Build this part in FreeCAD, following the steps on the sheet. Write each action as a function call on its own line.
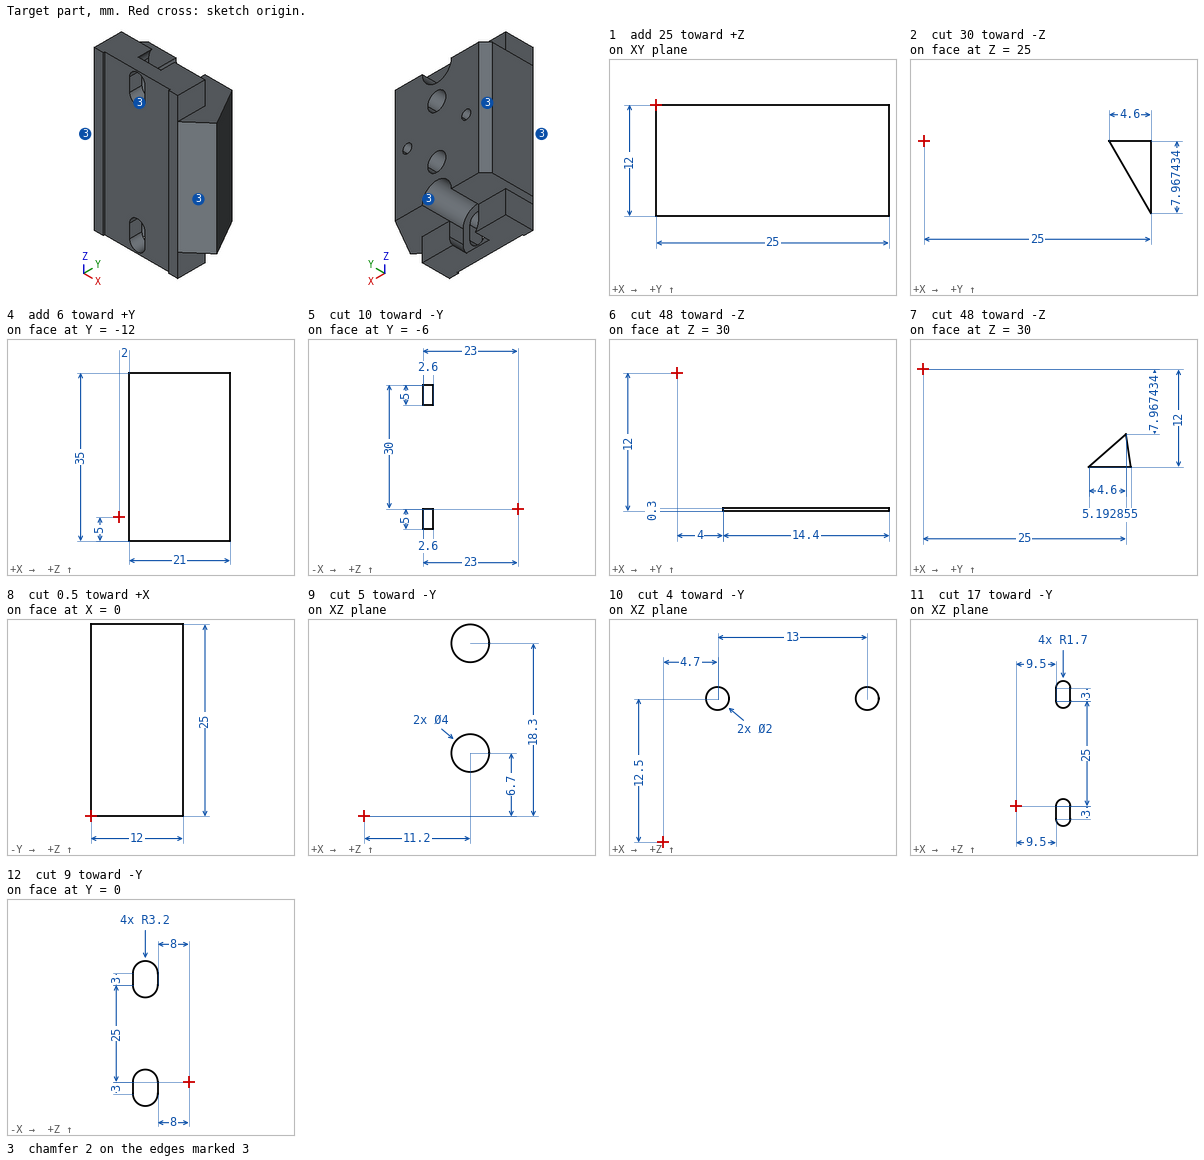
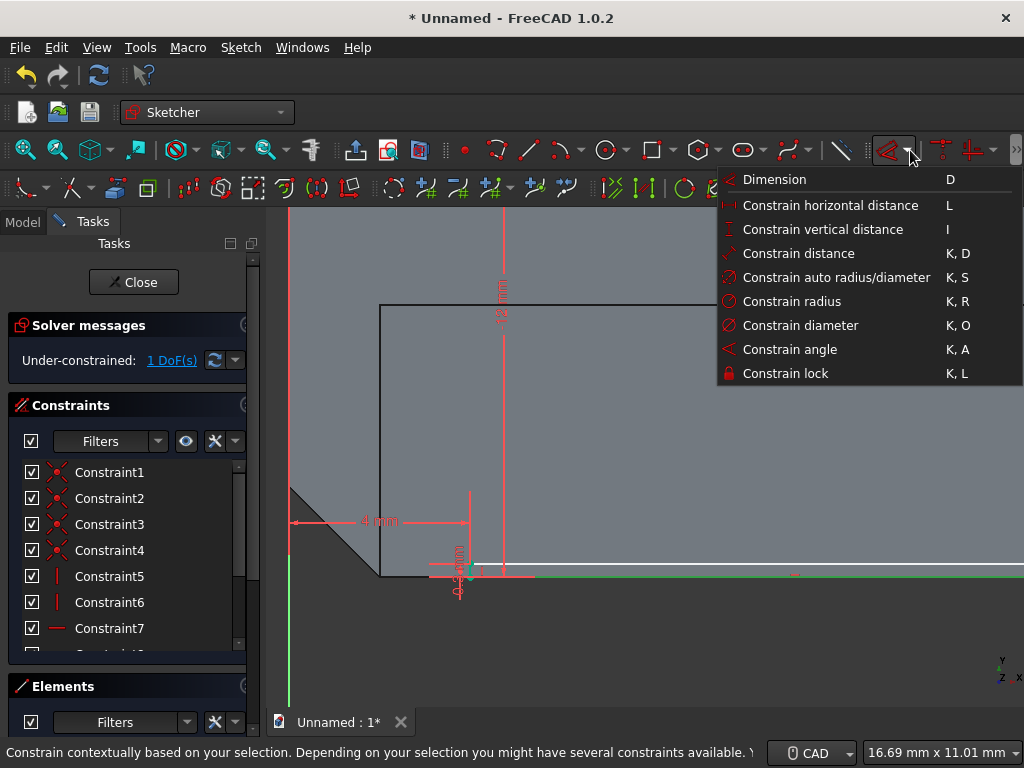
click(870, 205)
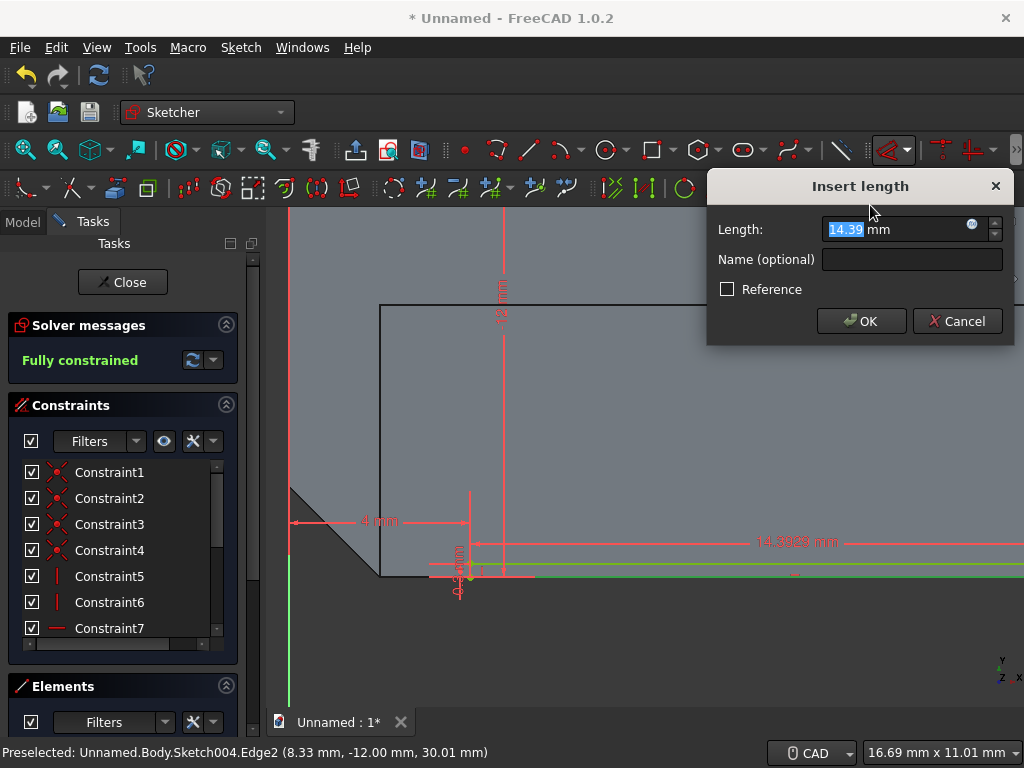
text(14.4)
key(Return)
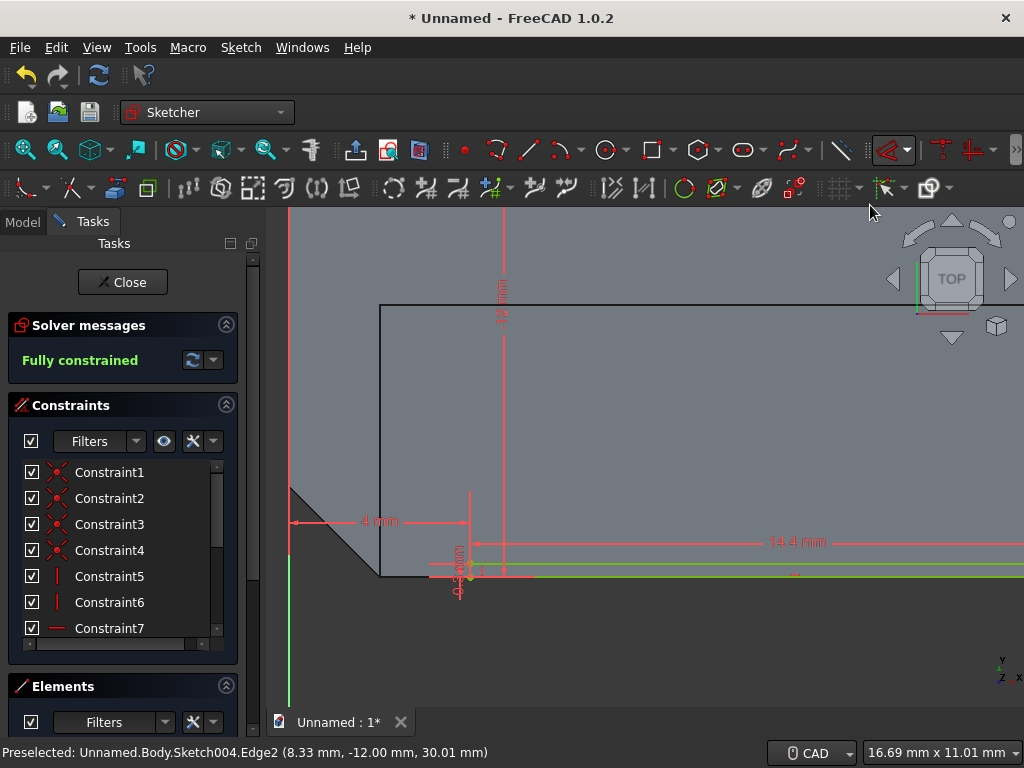
click(123, 282)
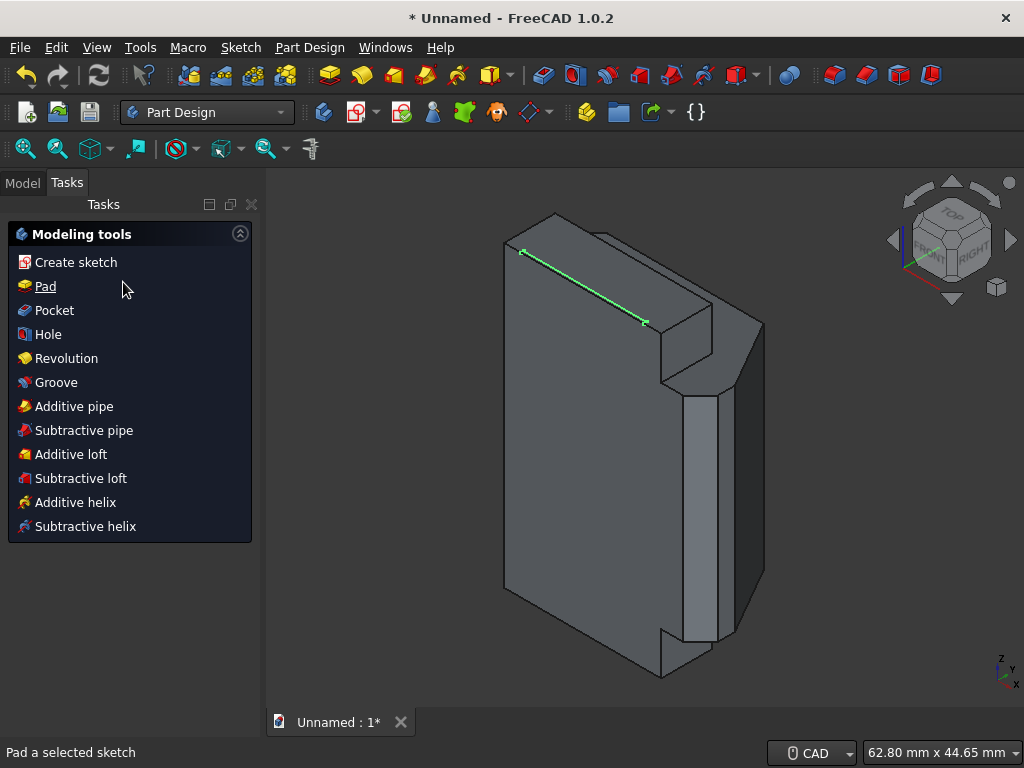
click(544, 76)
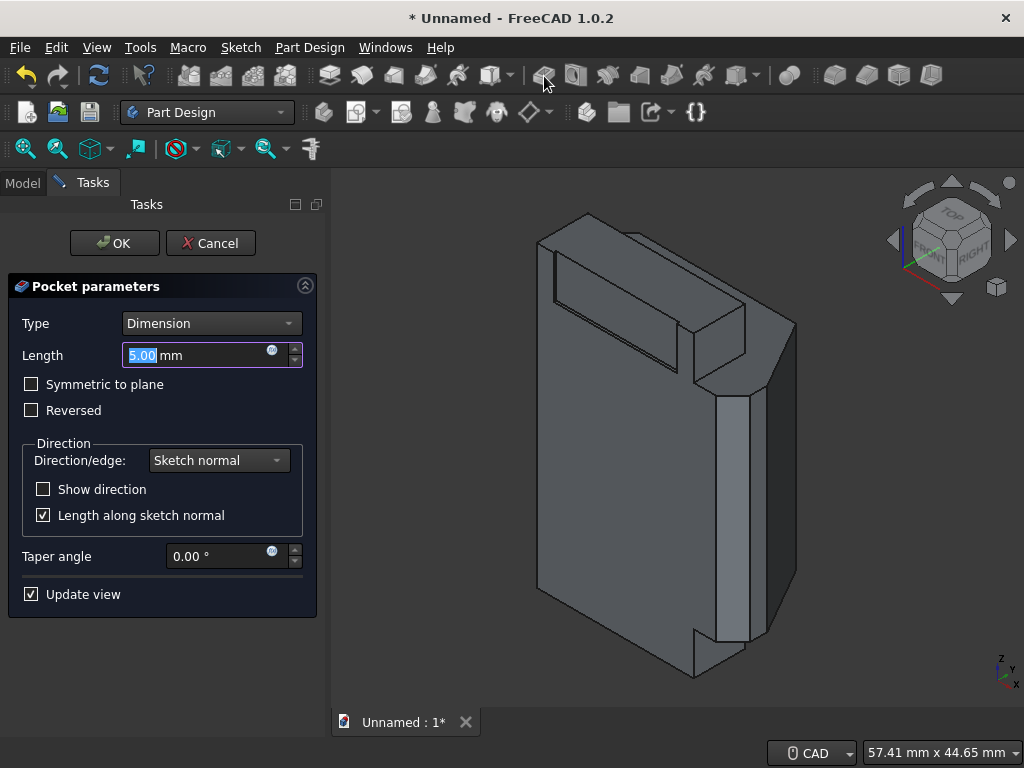
text(48)
key(Tab)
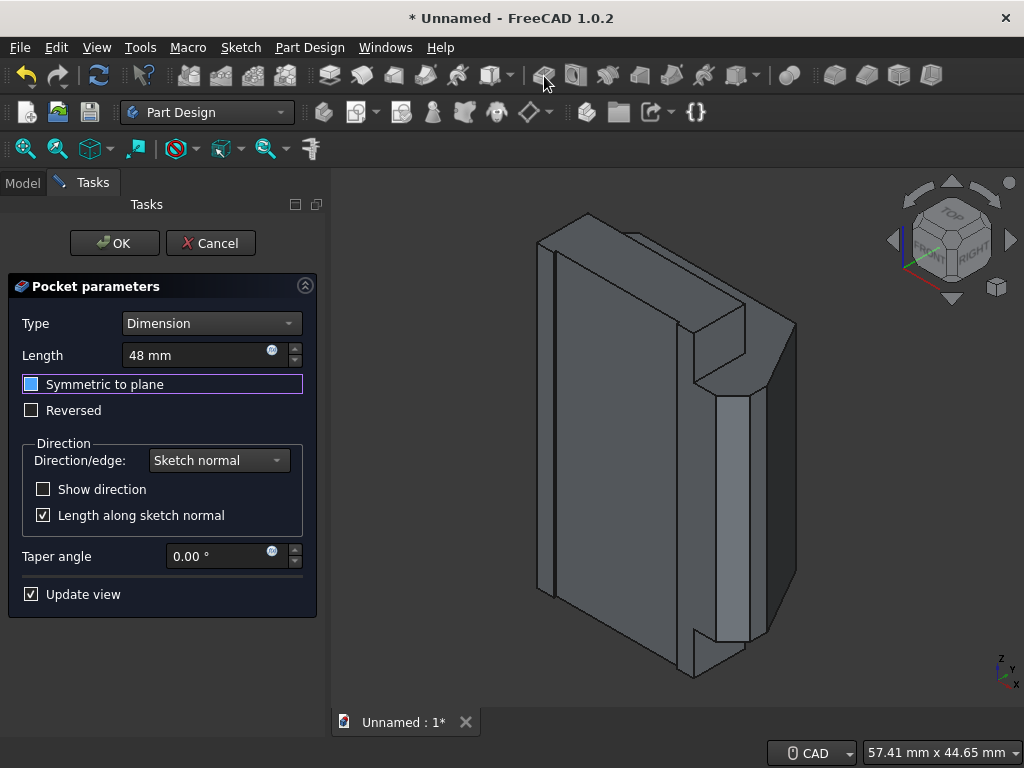
click(115, 243)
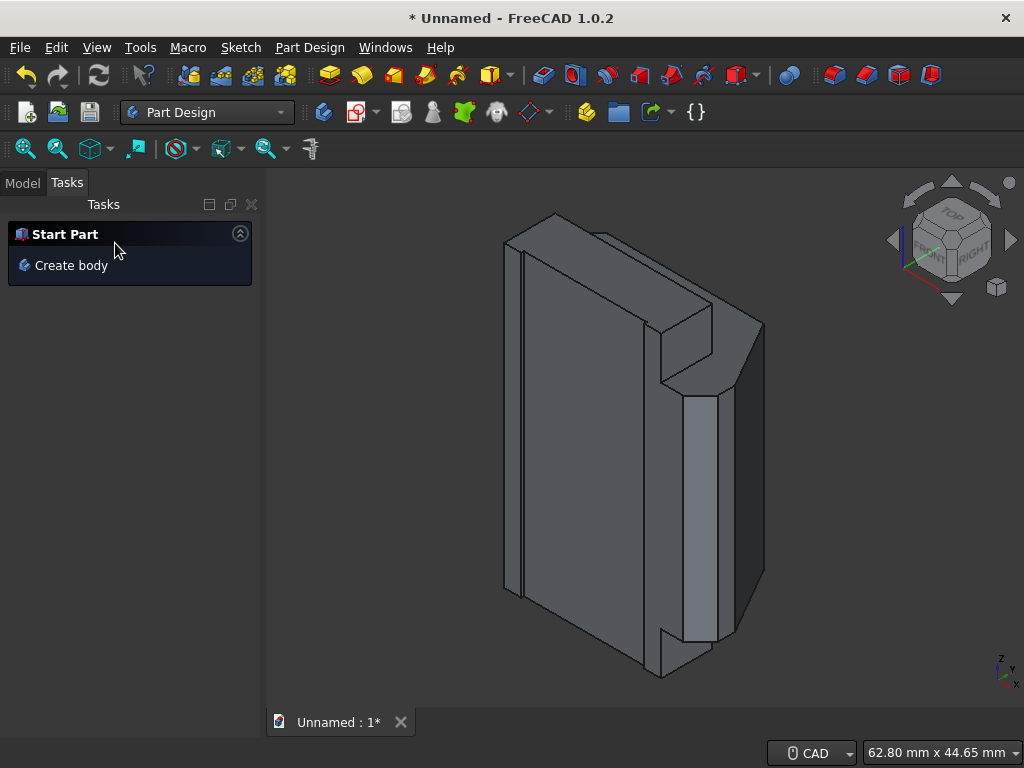
click(653, 298)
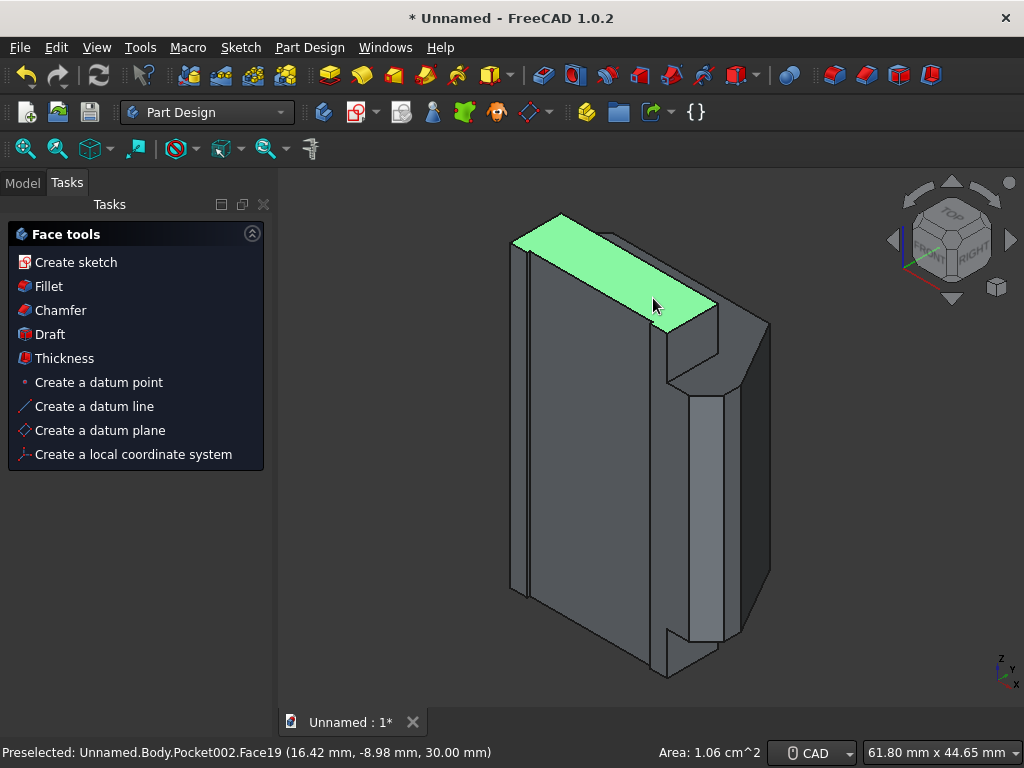
click(356, 112)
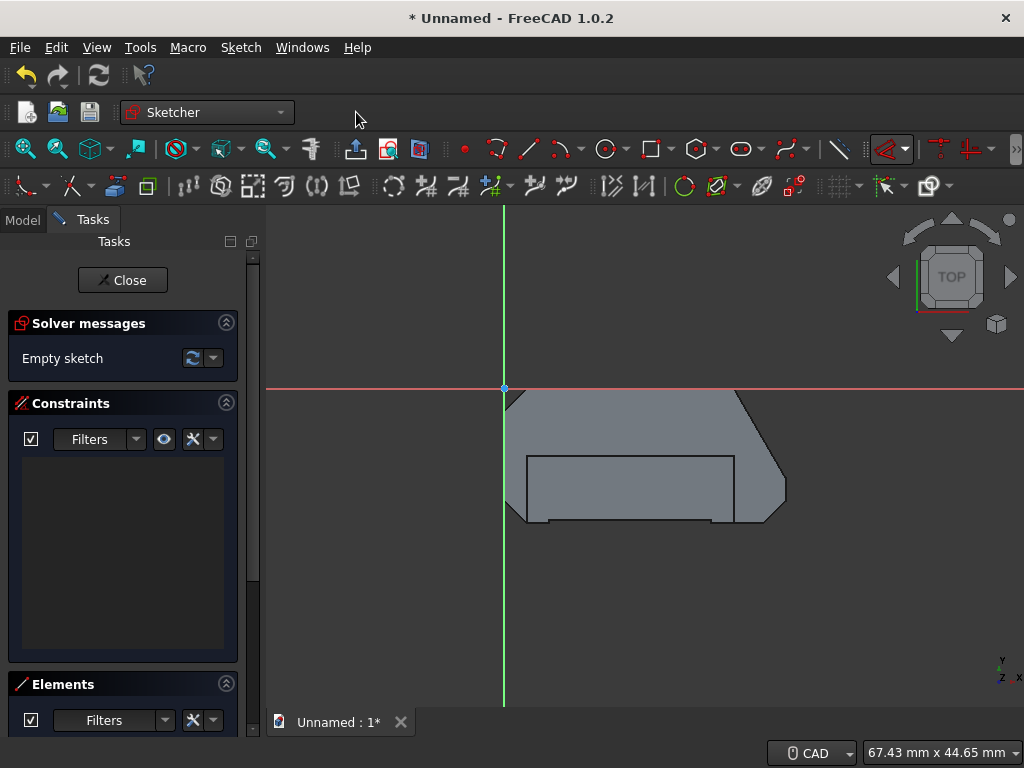
scroll(792, 508, up, 10)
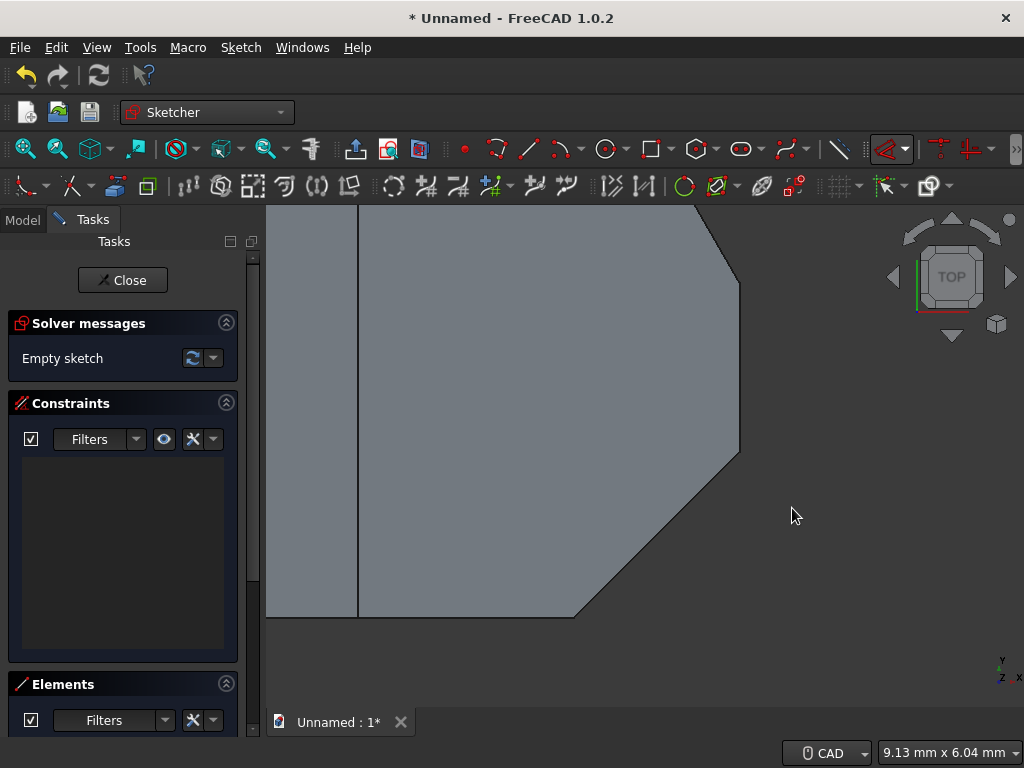
click(498, 150)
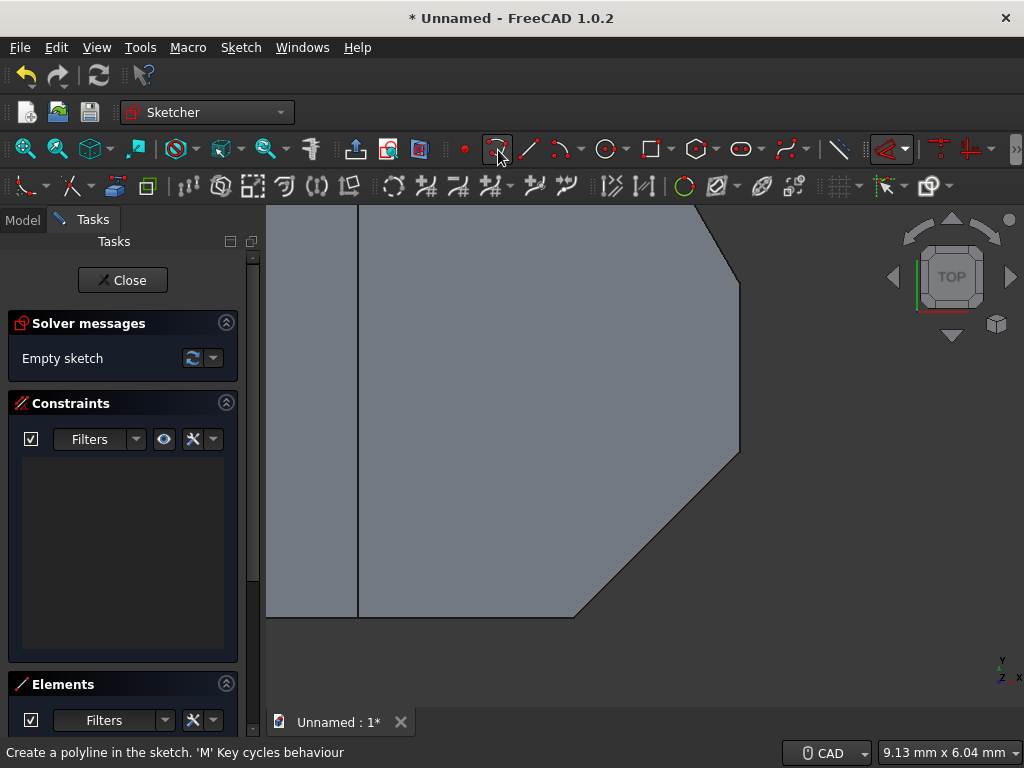
click(358, 618)
click(789, 618)
click(740, 283)
click(358, 619)
key(Escape)
key(Escape)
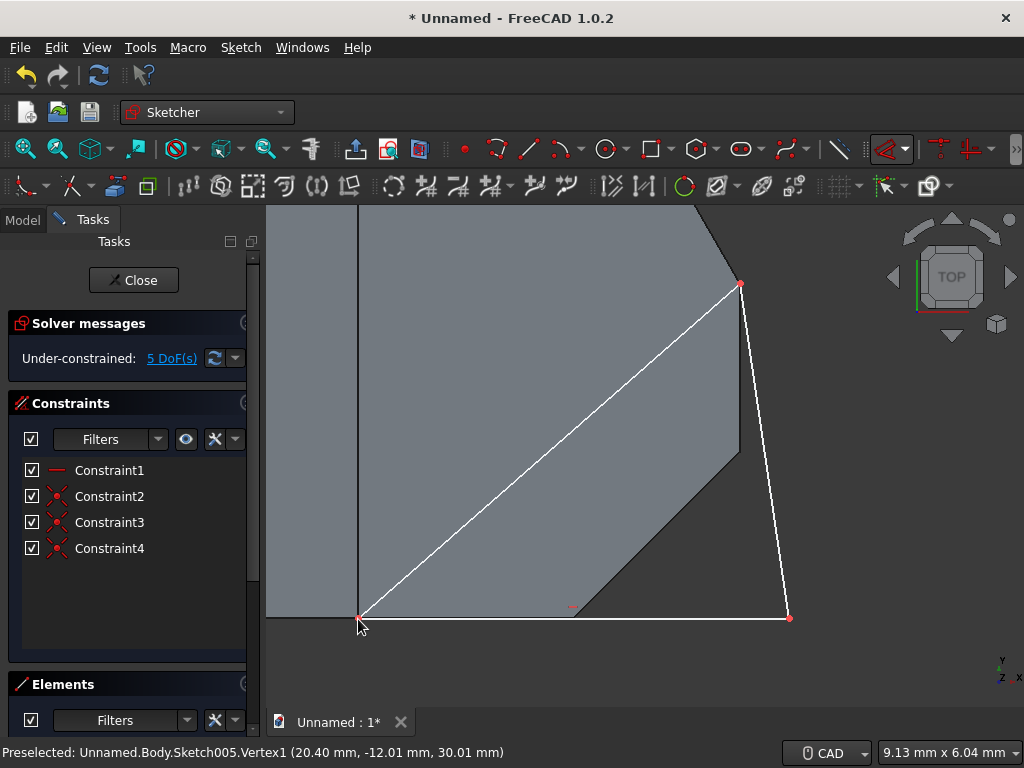
click(358, 619)